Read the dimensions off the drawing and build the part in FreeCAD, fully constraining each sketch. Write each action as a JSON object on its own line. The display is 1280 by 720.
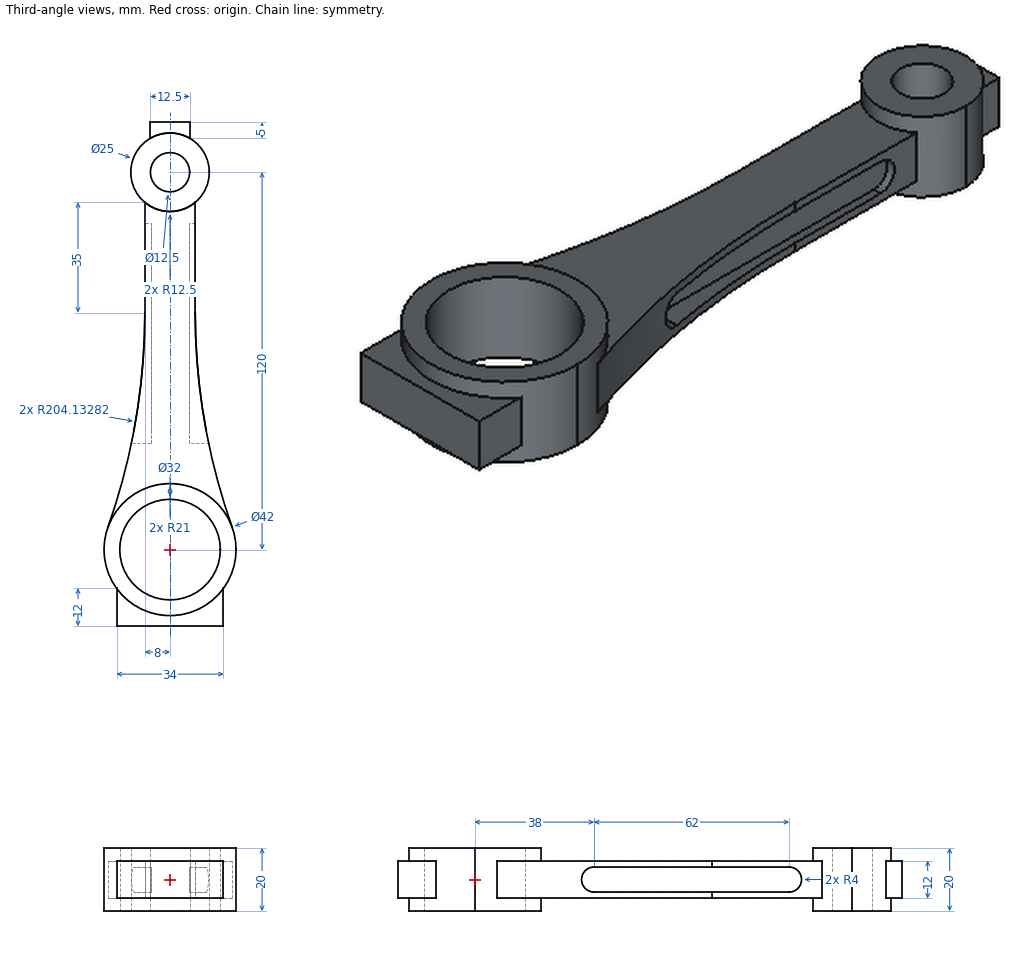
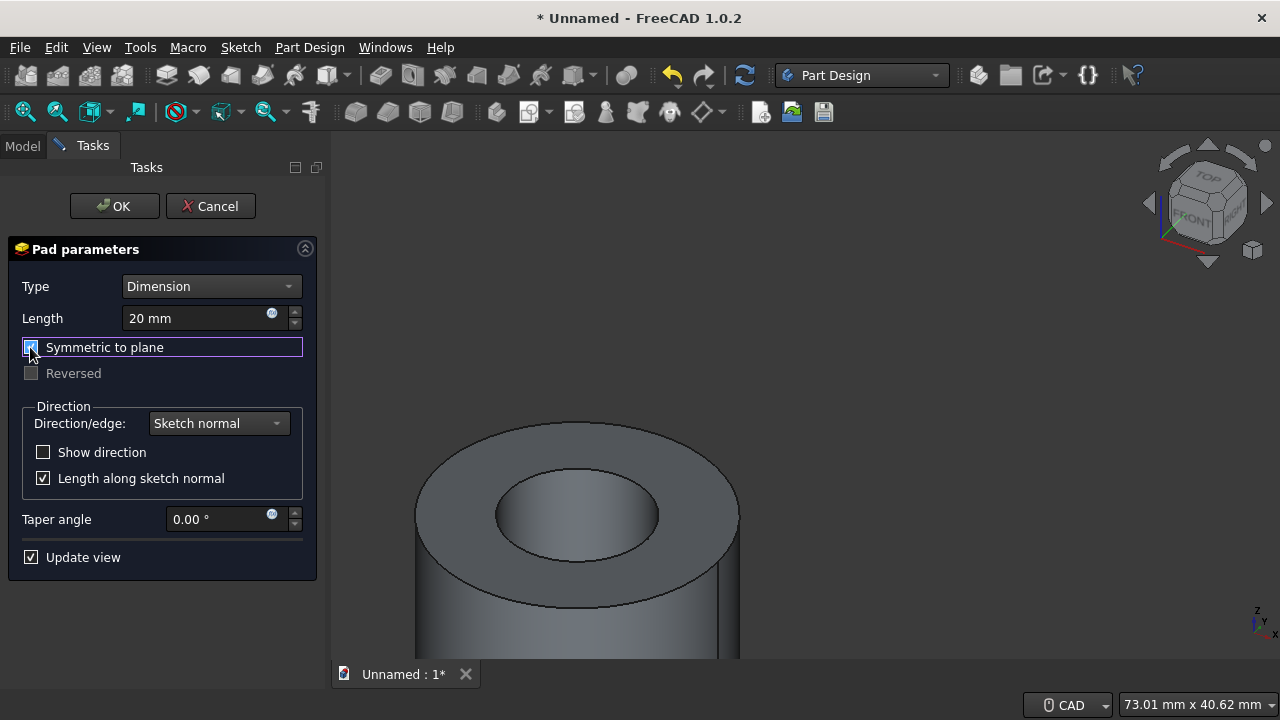
{"action": "left_click", "coordinate": [115, 206]}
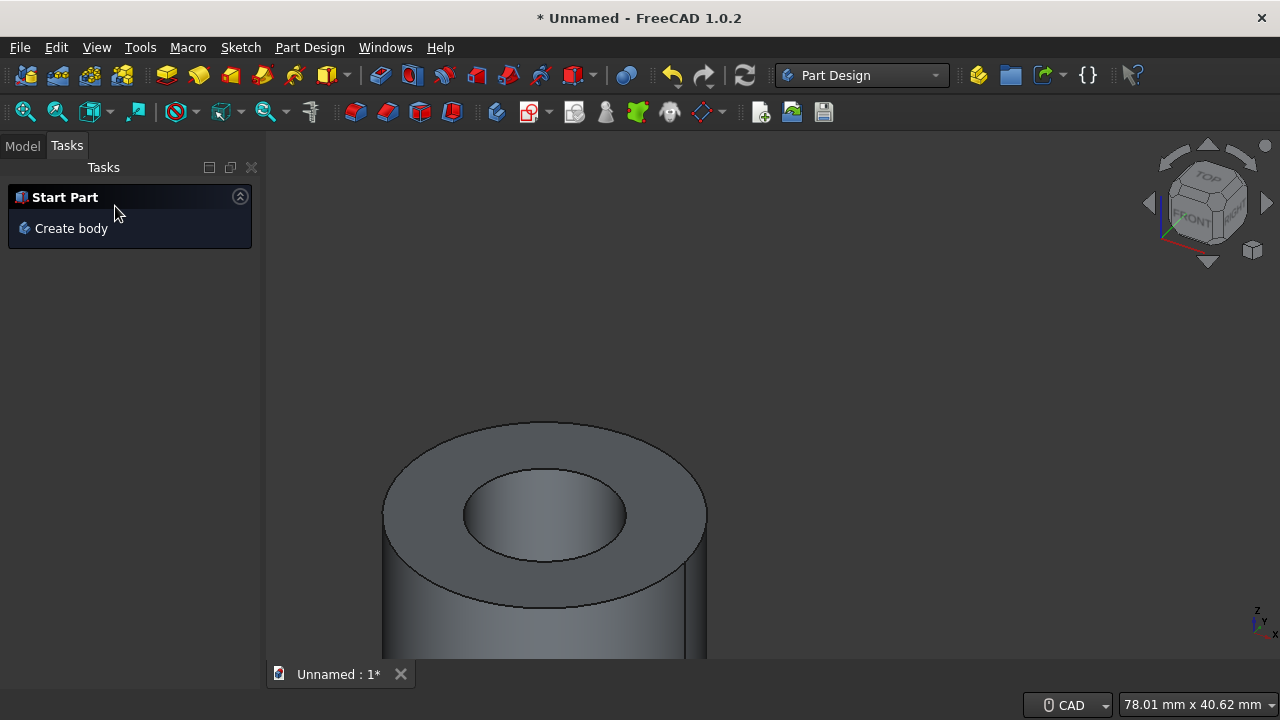
{"action": "key", "text": "v f"}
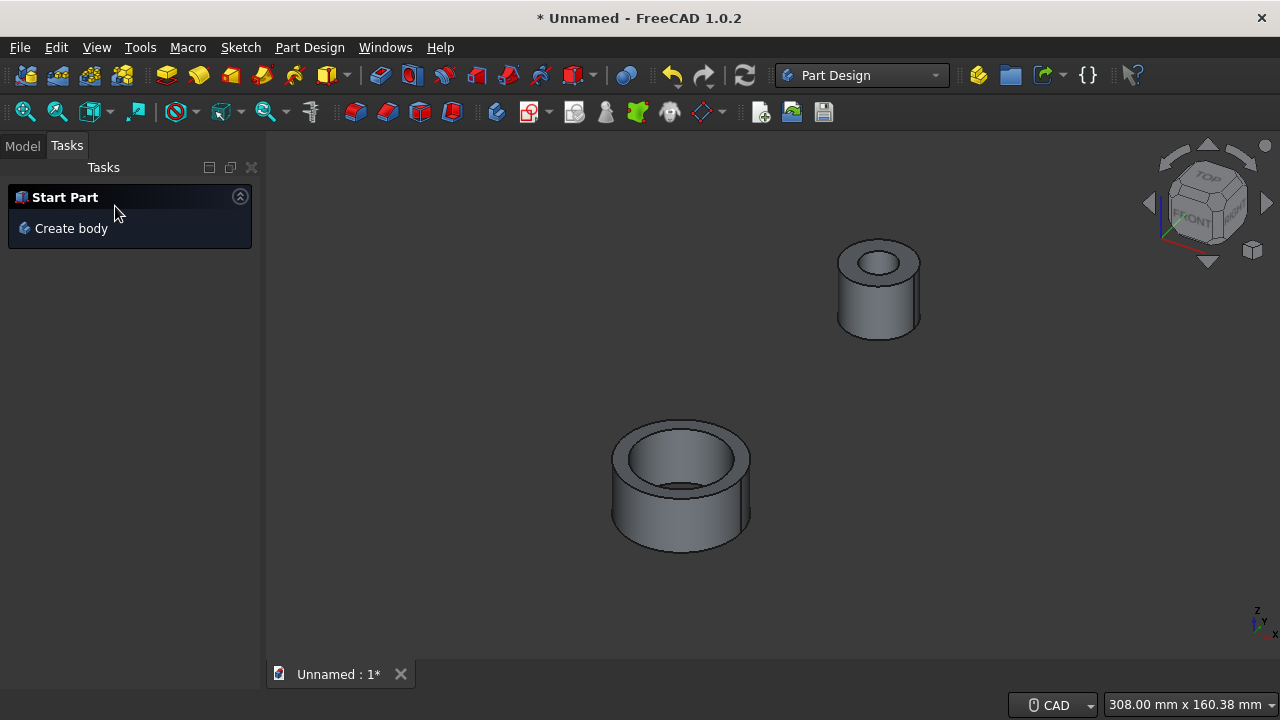
{"action": "left_click", "coordinate": [23, 145]}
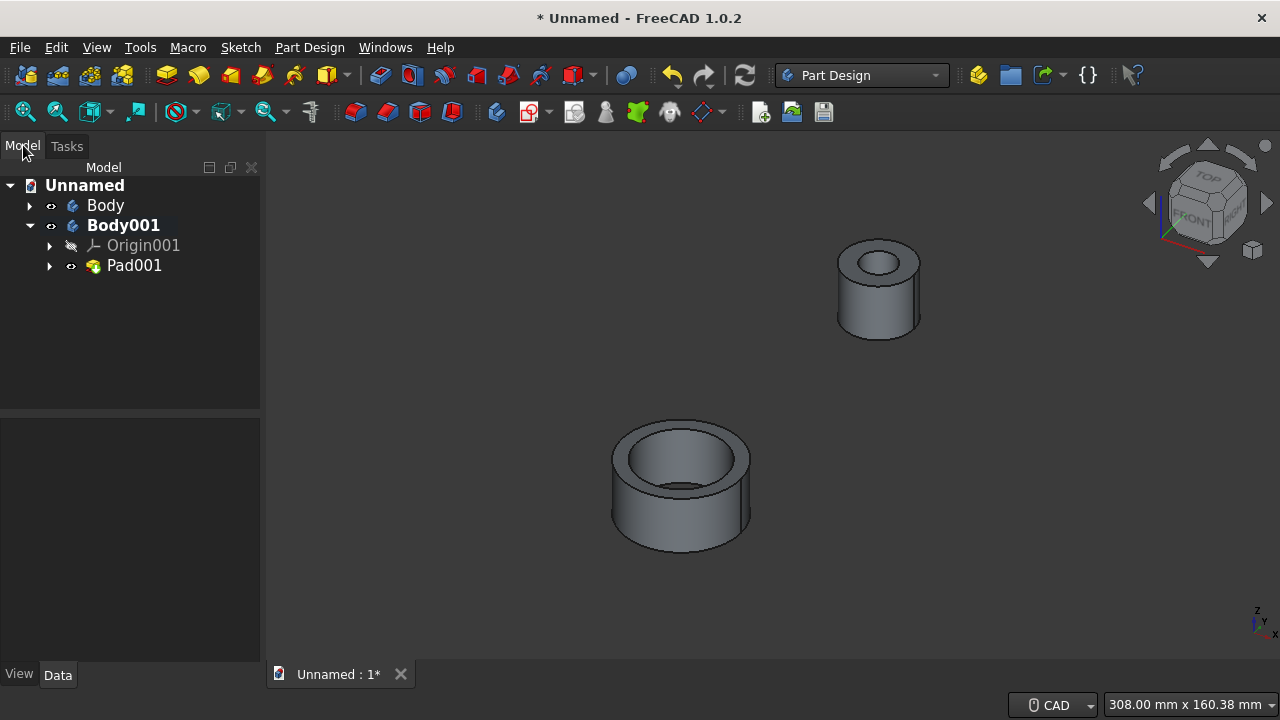
{"action": "double_click", "coordinate": [96, 206]}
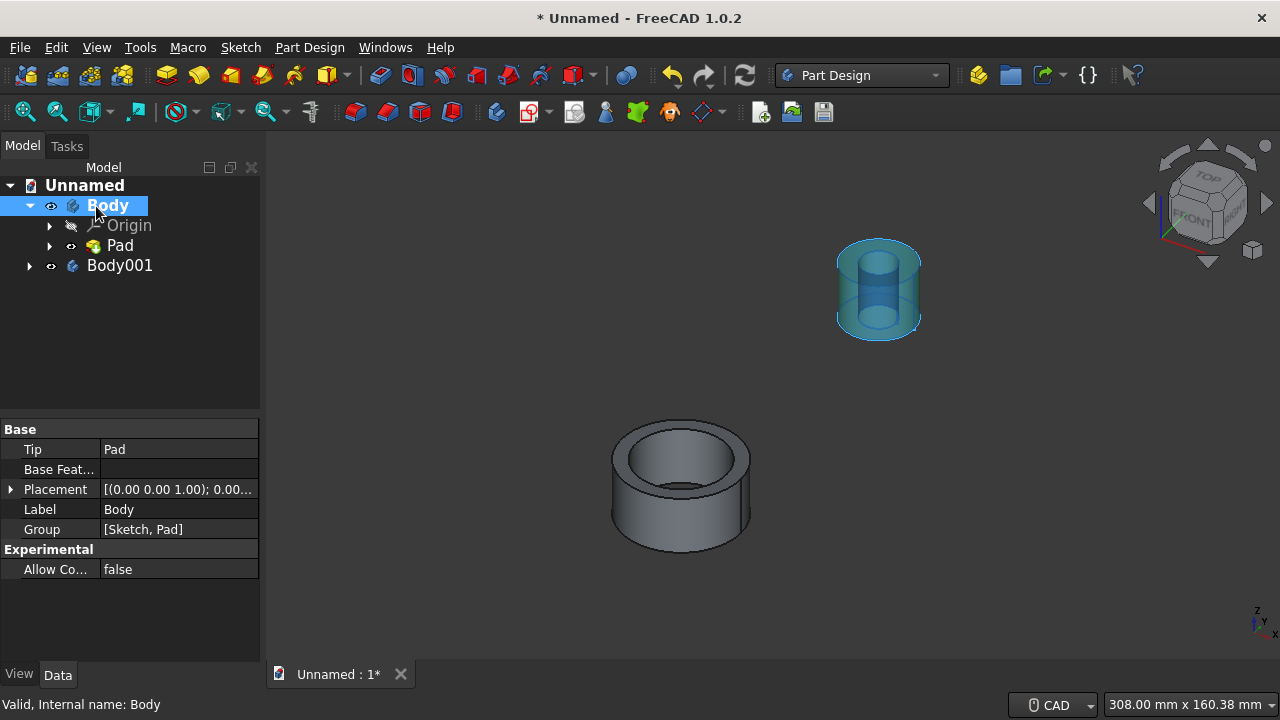
{"action": "left_click", "coordinate": [96, 206]}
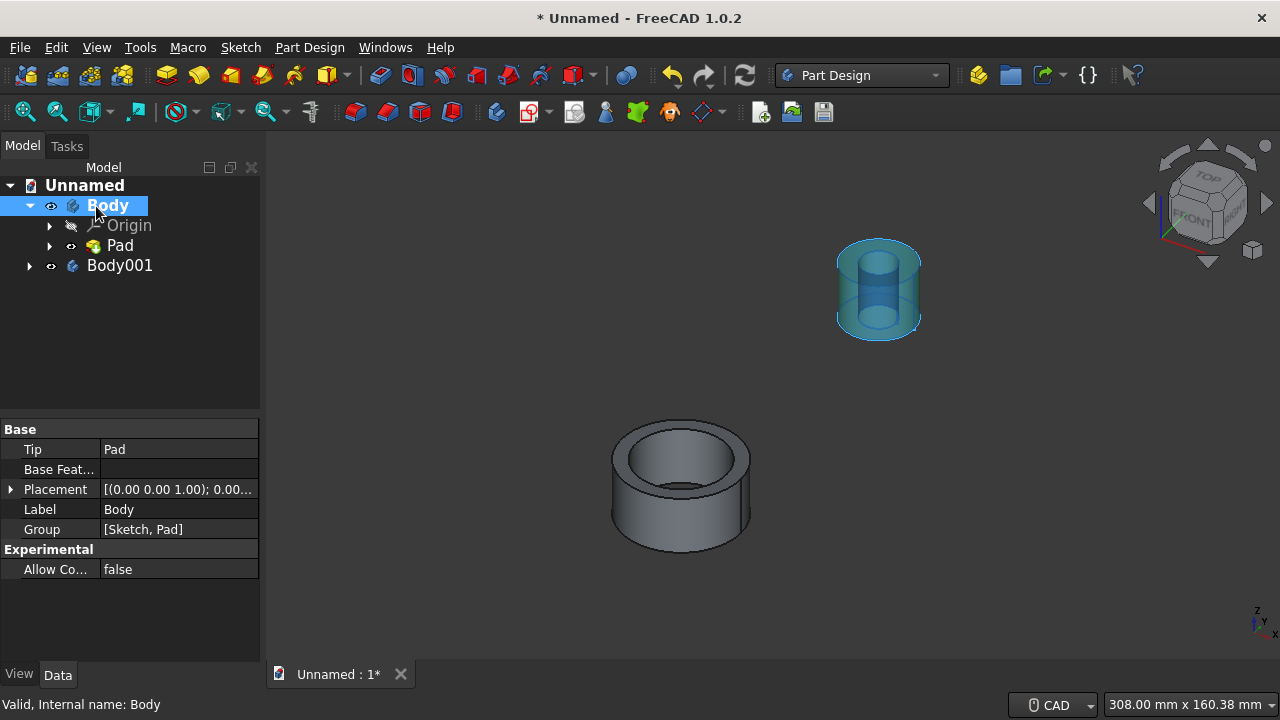
{"action": "left_click", "coordinate": [146, 569]}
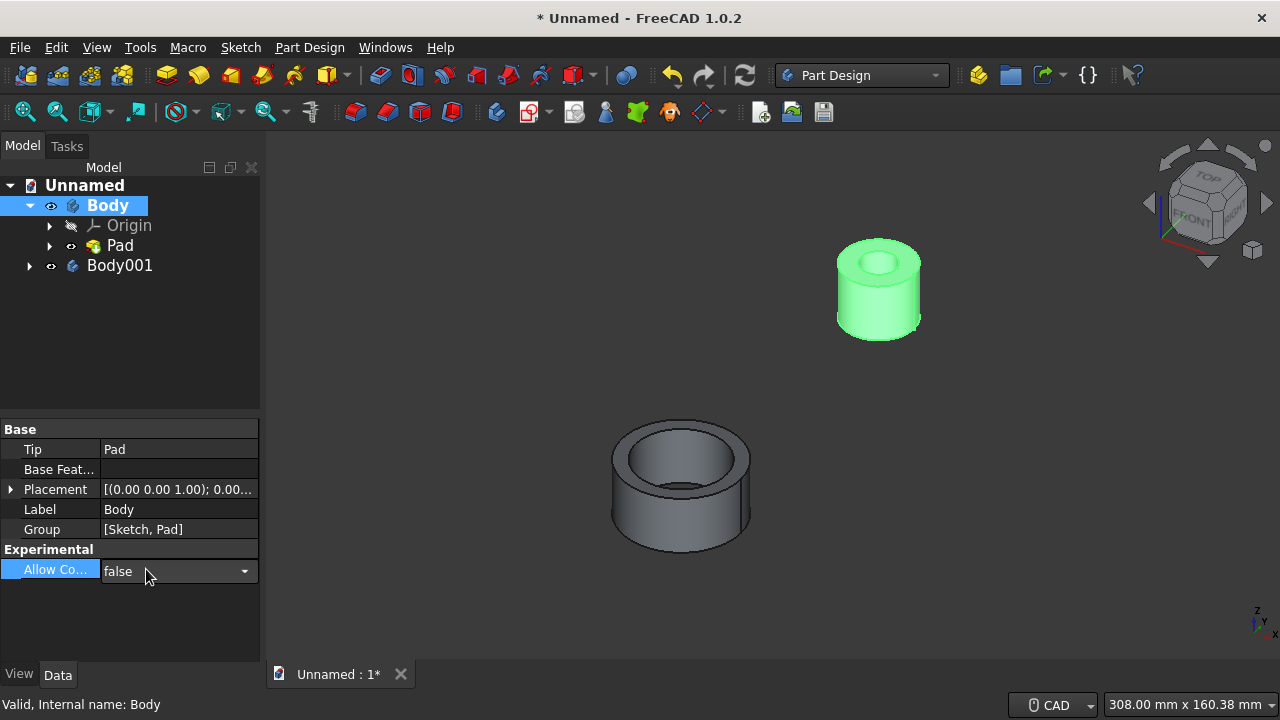
{"action": "left_click", "coordinate": [146, 569]}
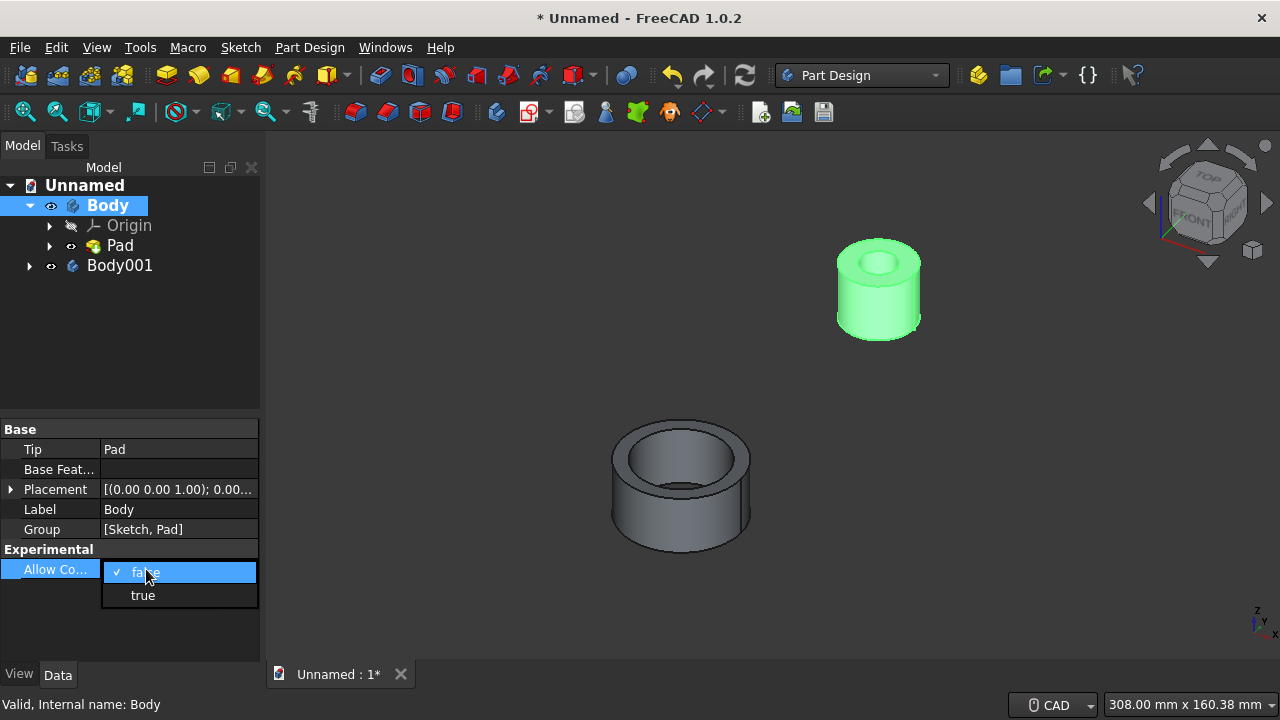
{"action": "left_click", "coordinate": [179, 596]}
{"action": "key", "text": "Return"}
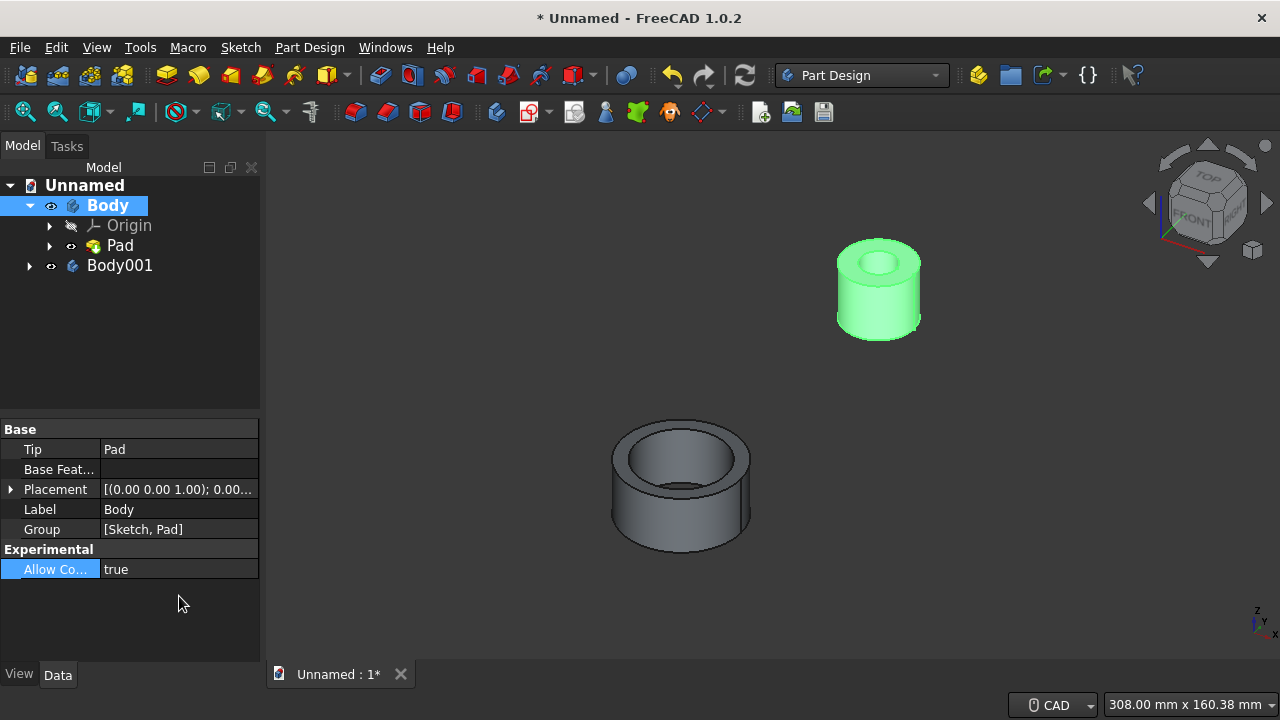
{"action": "left_click", "coordinate": [96, 266]}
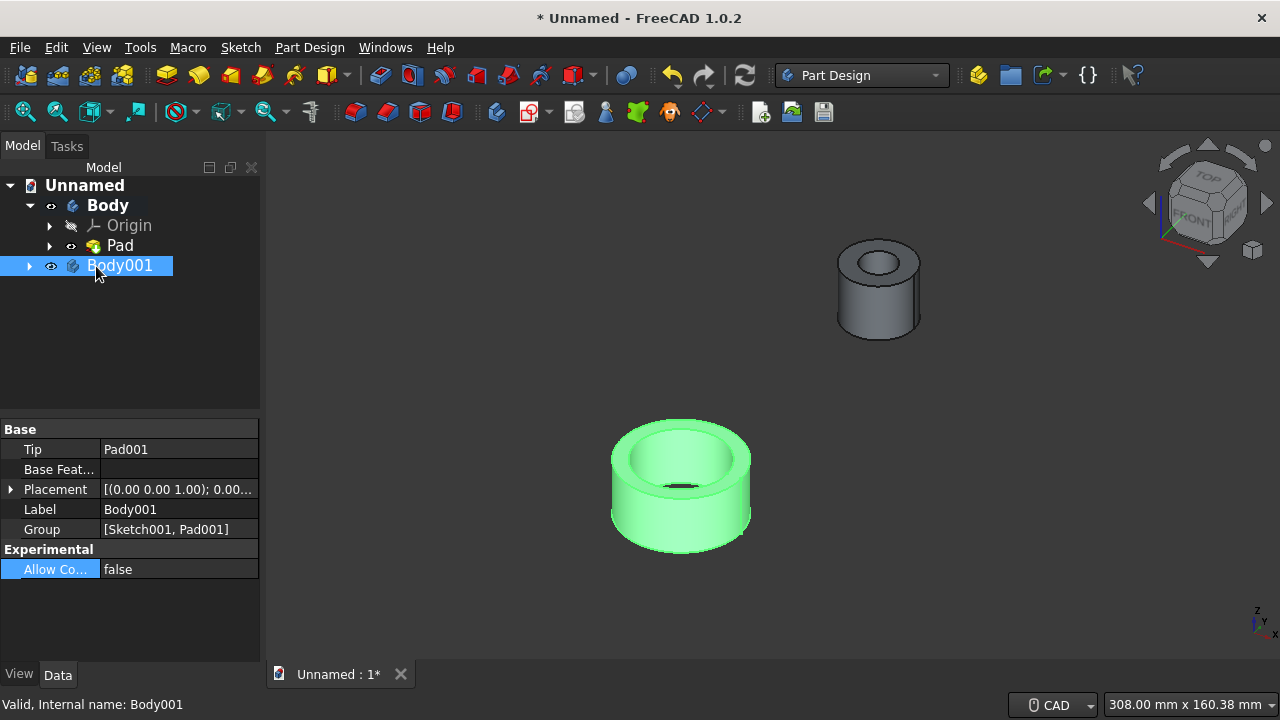
{"action": "left_click", "coordinate": [628, 76]}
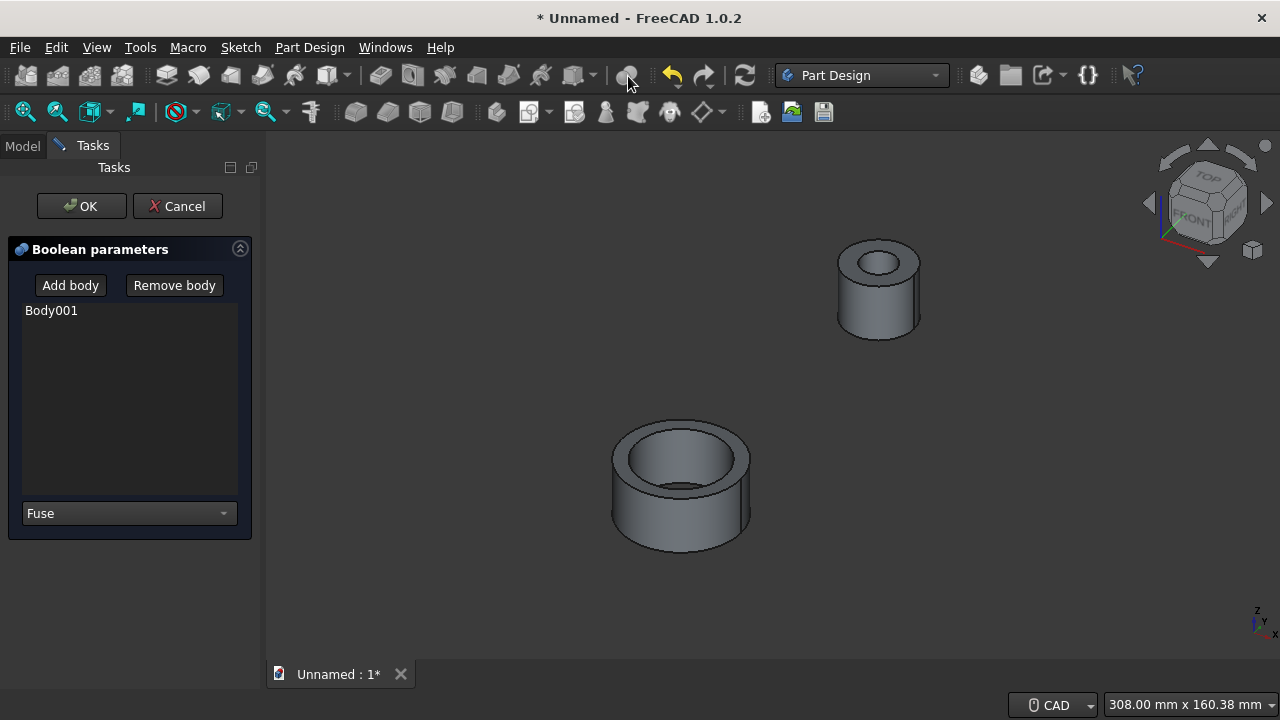
{"action": "left_click", "coordinate": [82, 206]}